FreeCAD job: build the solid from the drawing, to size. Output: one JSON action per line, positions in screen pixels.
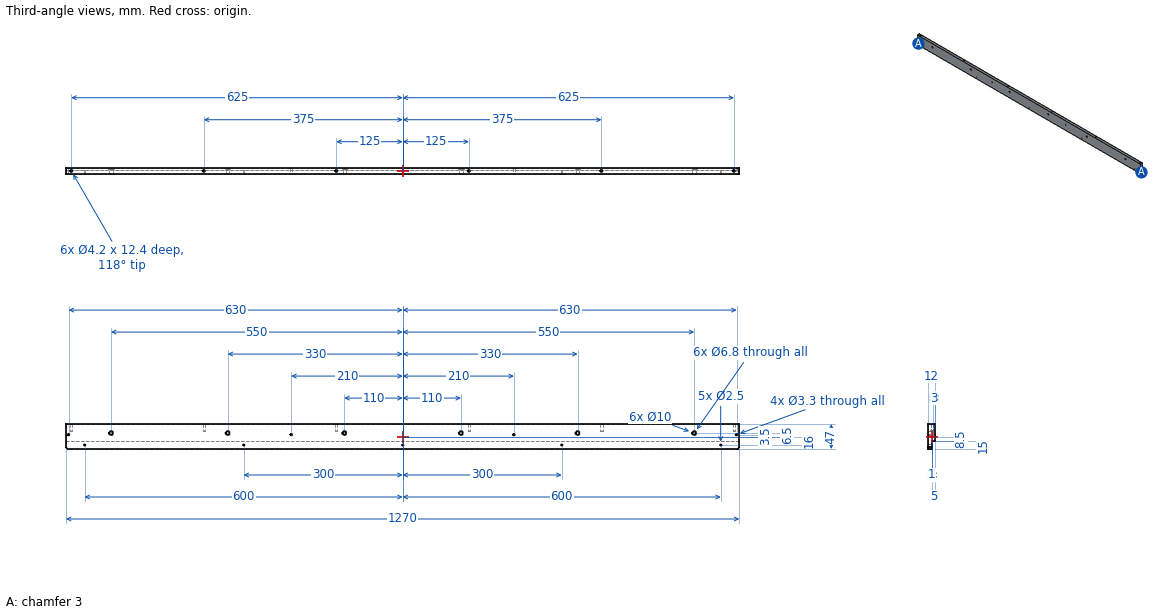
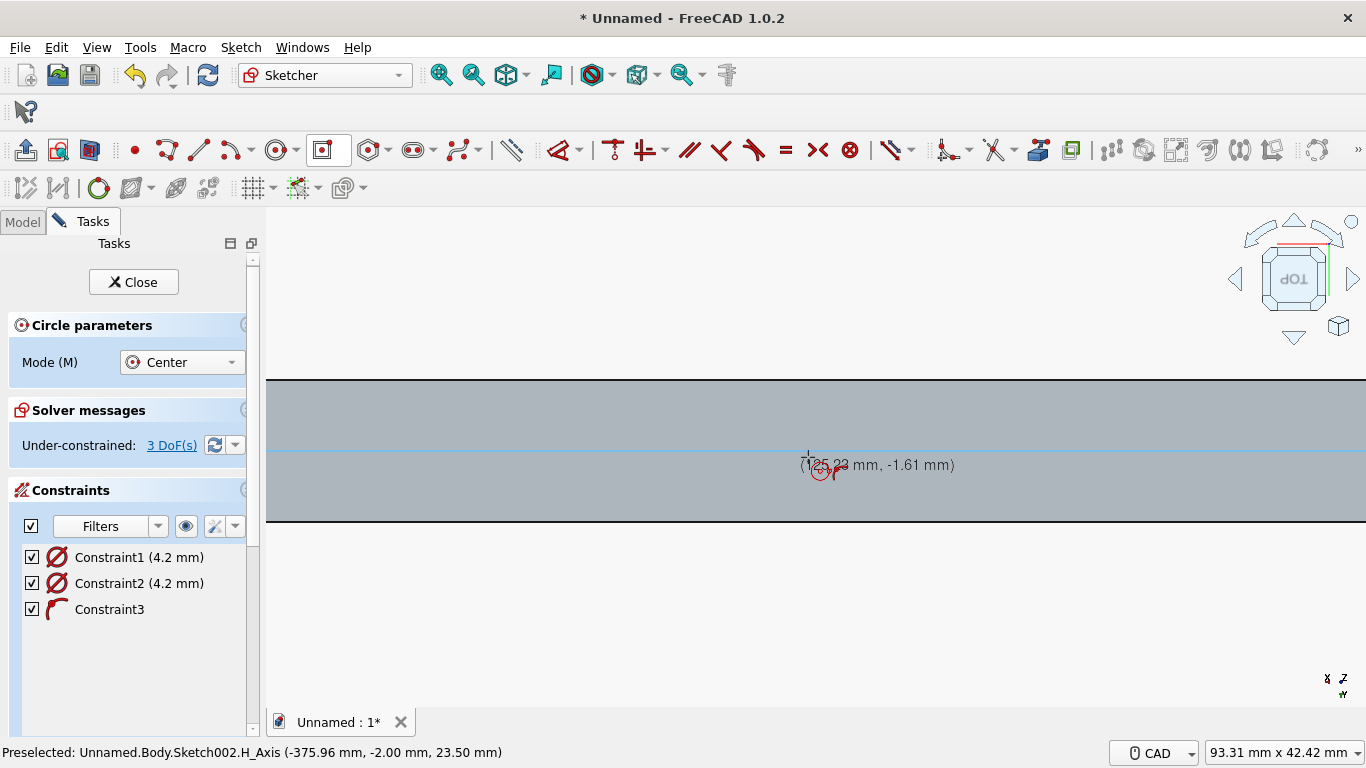
{"action": "scroll", "coordinate": [822, 457], "scroll_direction": "down", "scroll_amount": 15}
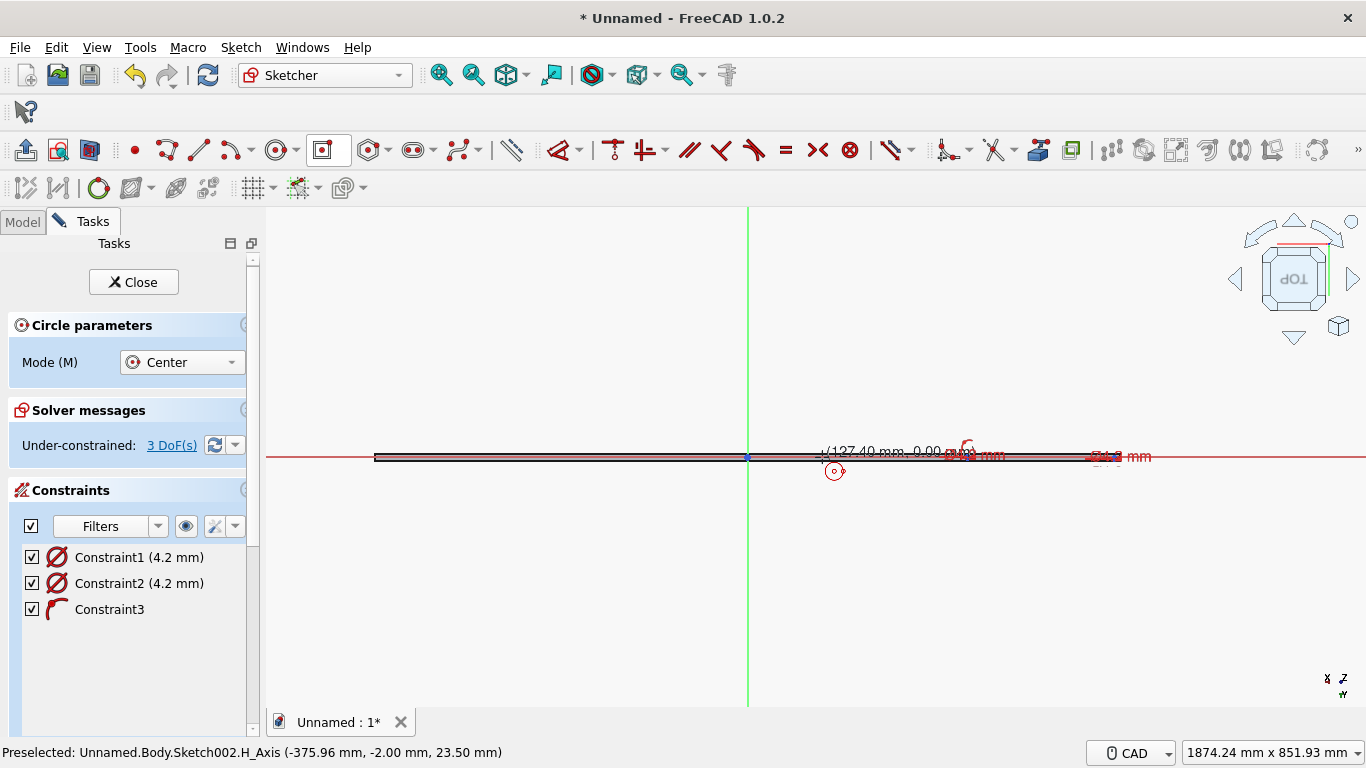
{"action": "left_click", "coordinate": [821, 457]}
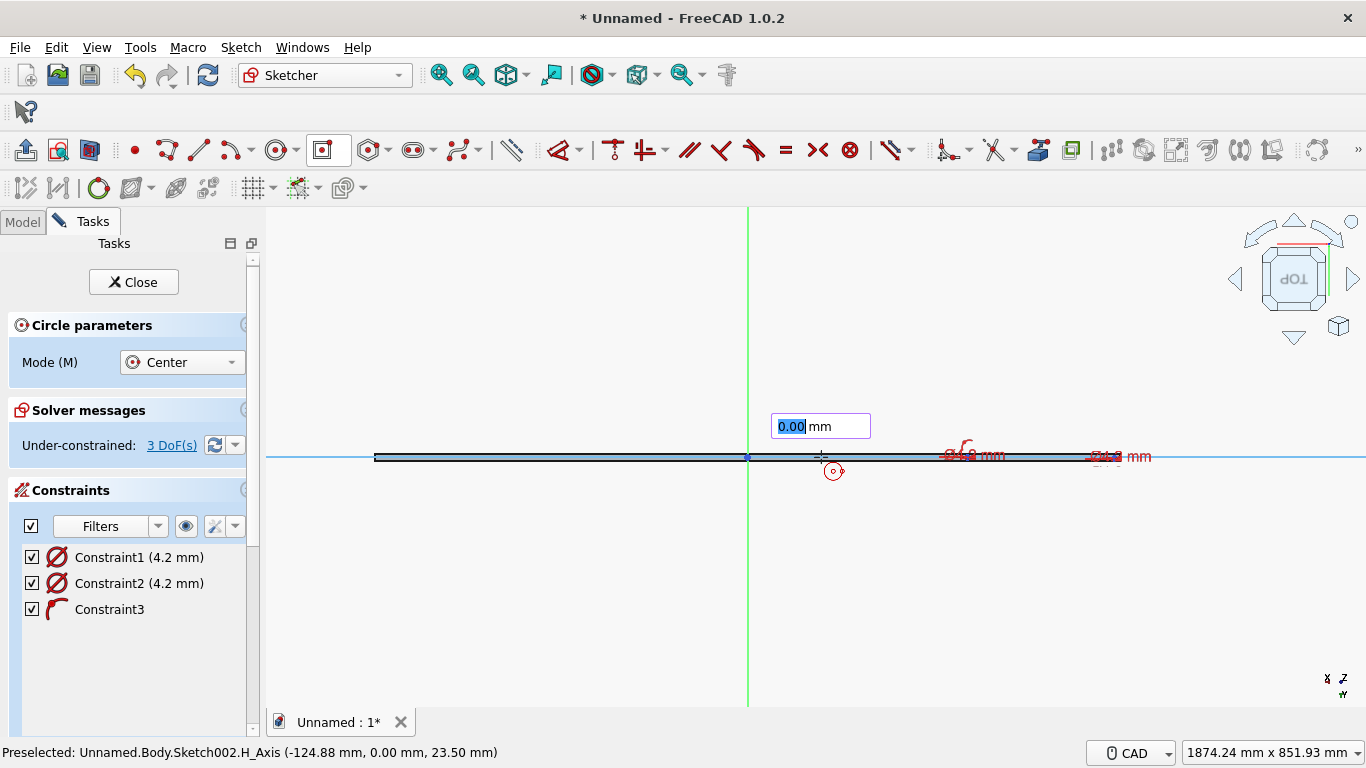
{"action": "scroll", "coordinate": [821, 458], "scroll_direction": "up", "scroll_amount": 14}
{"action": "mouse_move", "coordinate": [807, 456]}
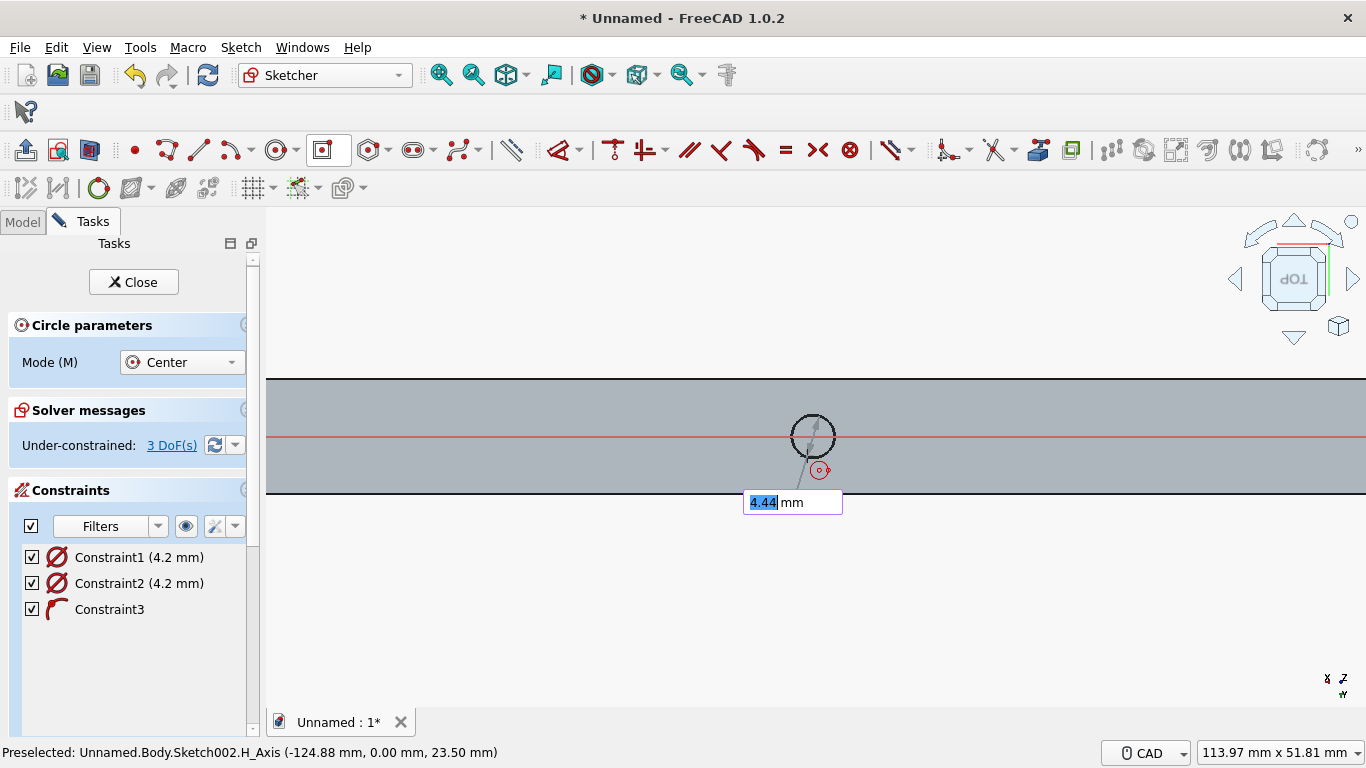
{"action": "type", "text": "4.2"}
{"action": "key", "text": "Return"}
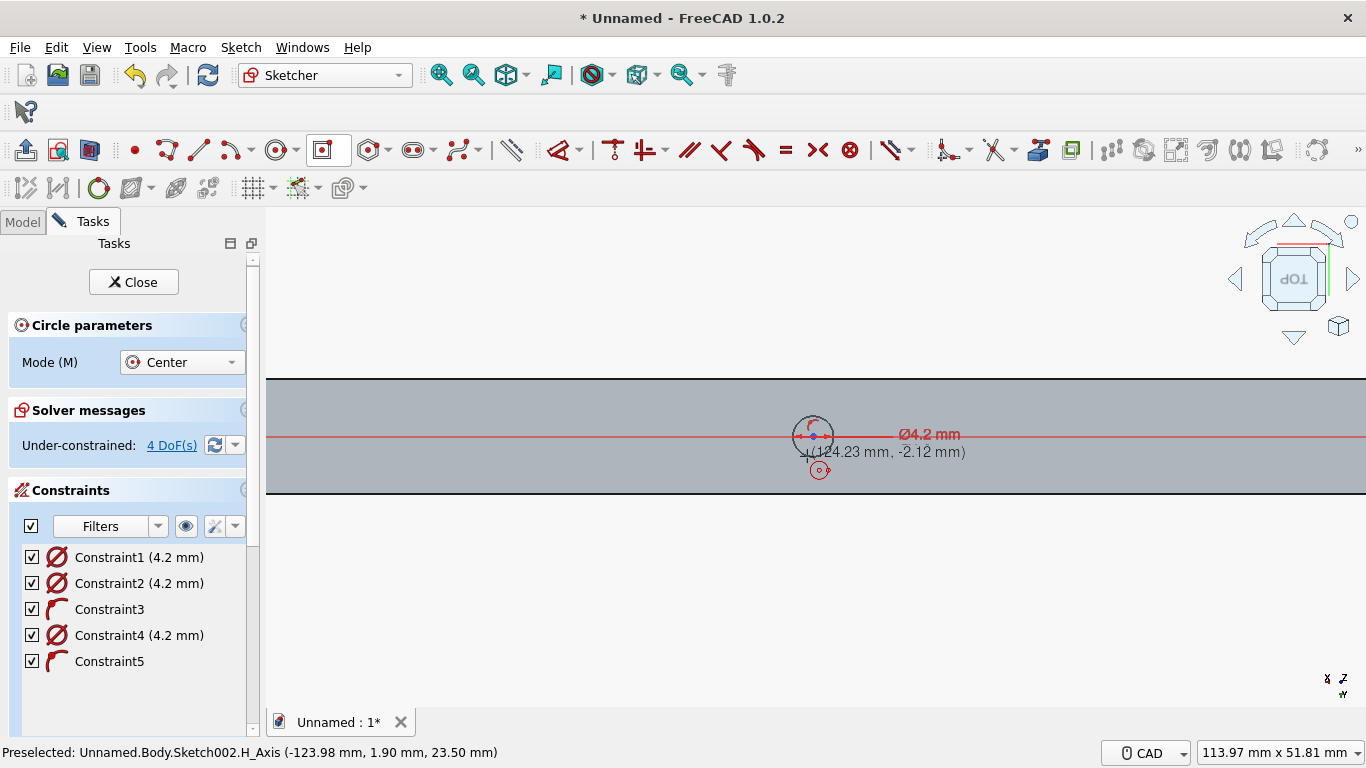
{"action": "scroll", "coordinate": [807, 458], "scroll_direction": "down", "scroll_amount": 15}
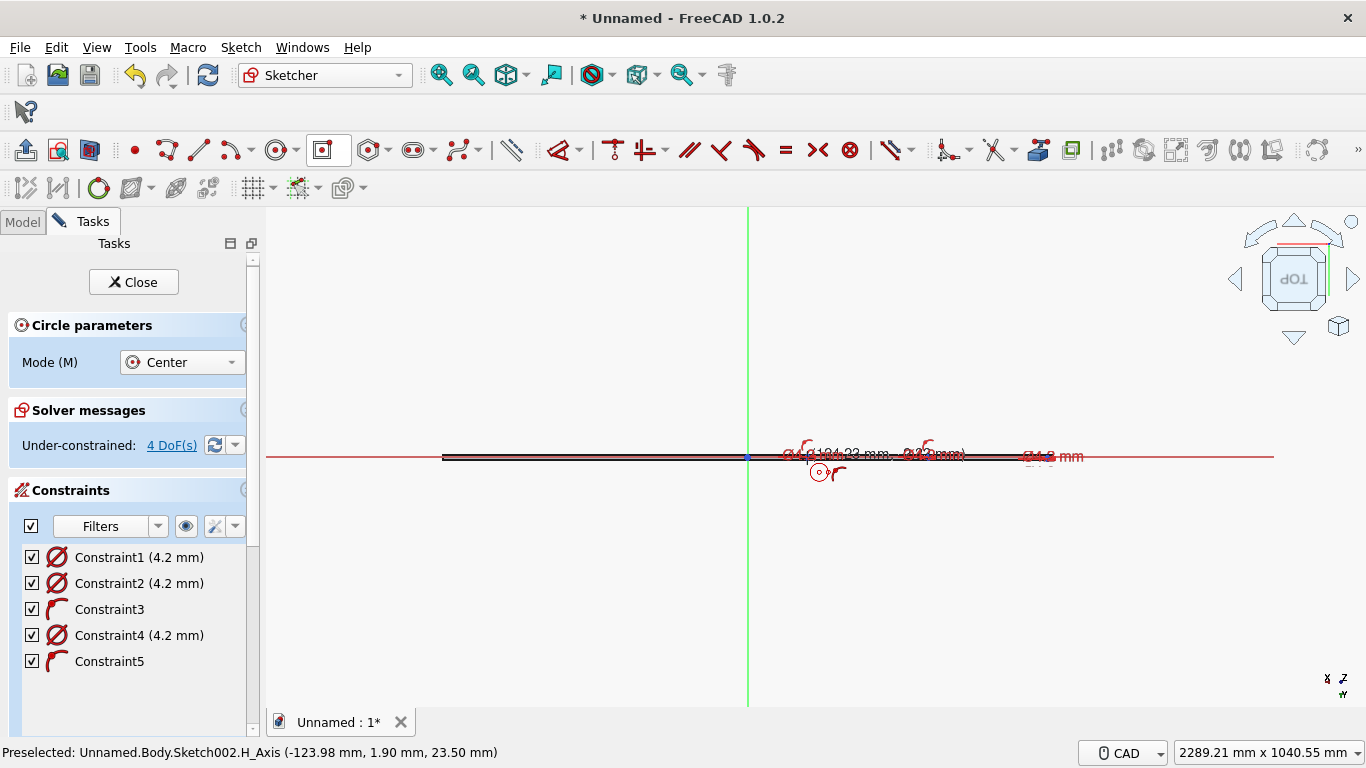
{"action": "scroll", "coordinate": [688, 457], "scroll_direction": "up", "scroll_amount": 16}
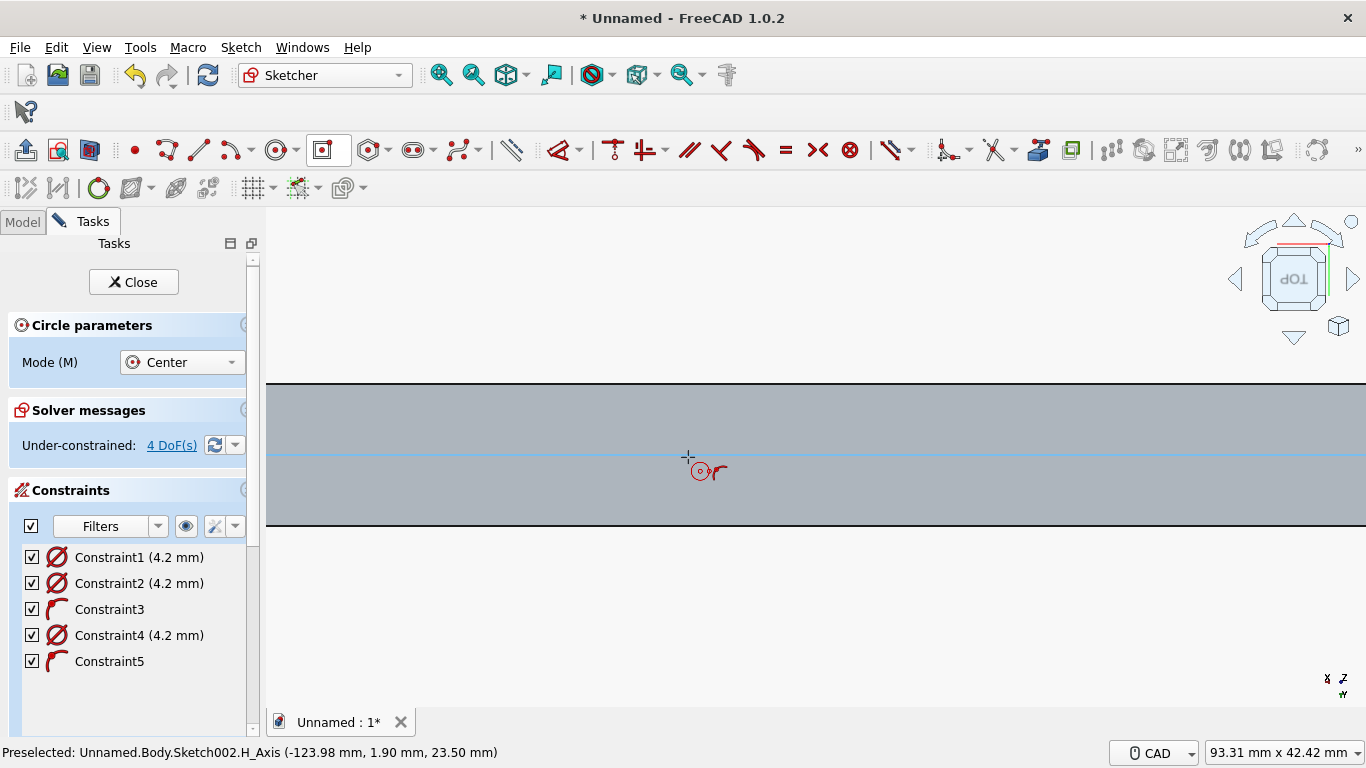
{"action": "scroll", "coordinate": [674, 457], "scroll_direction": "down", "scroll_amount": 15}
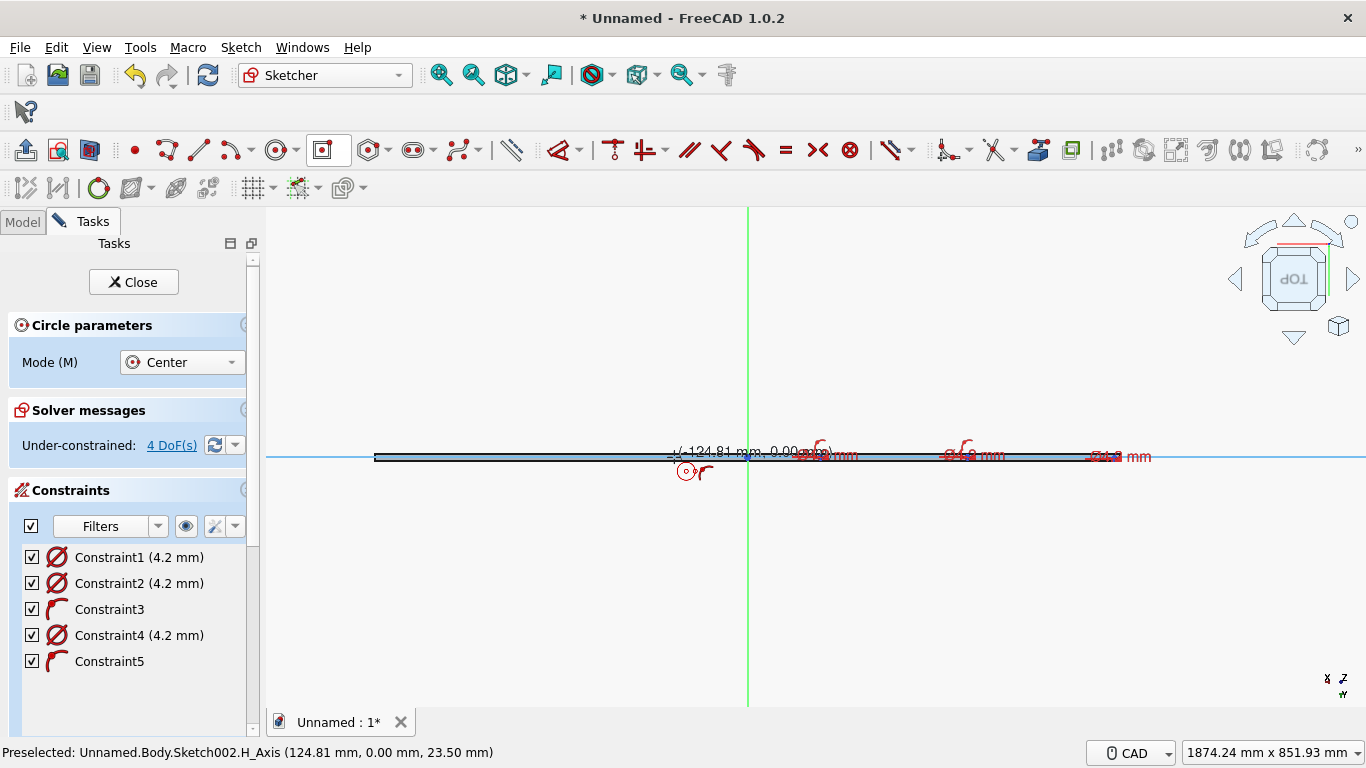
{"action": "left_click", "coordinate": [674, 457]}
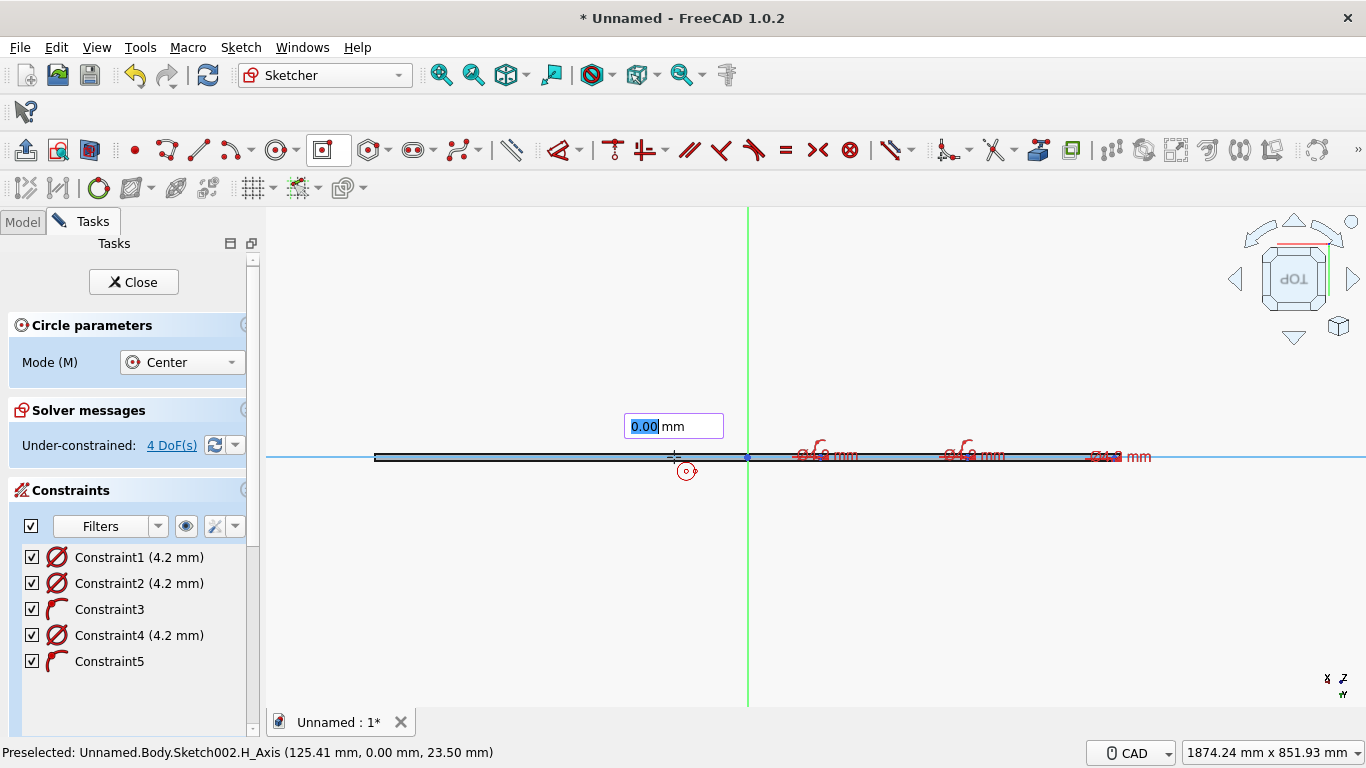
{"action": "scroll", "coordinate": [674, 459], "scroll_direction": "up", "scroll_amount": 14}
{"action": "mouse_move", "coordinate": [665, 444]}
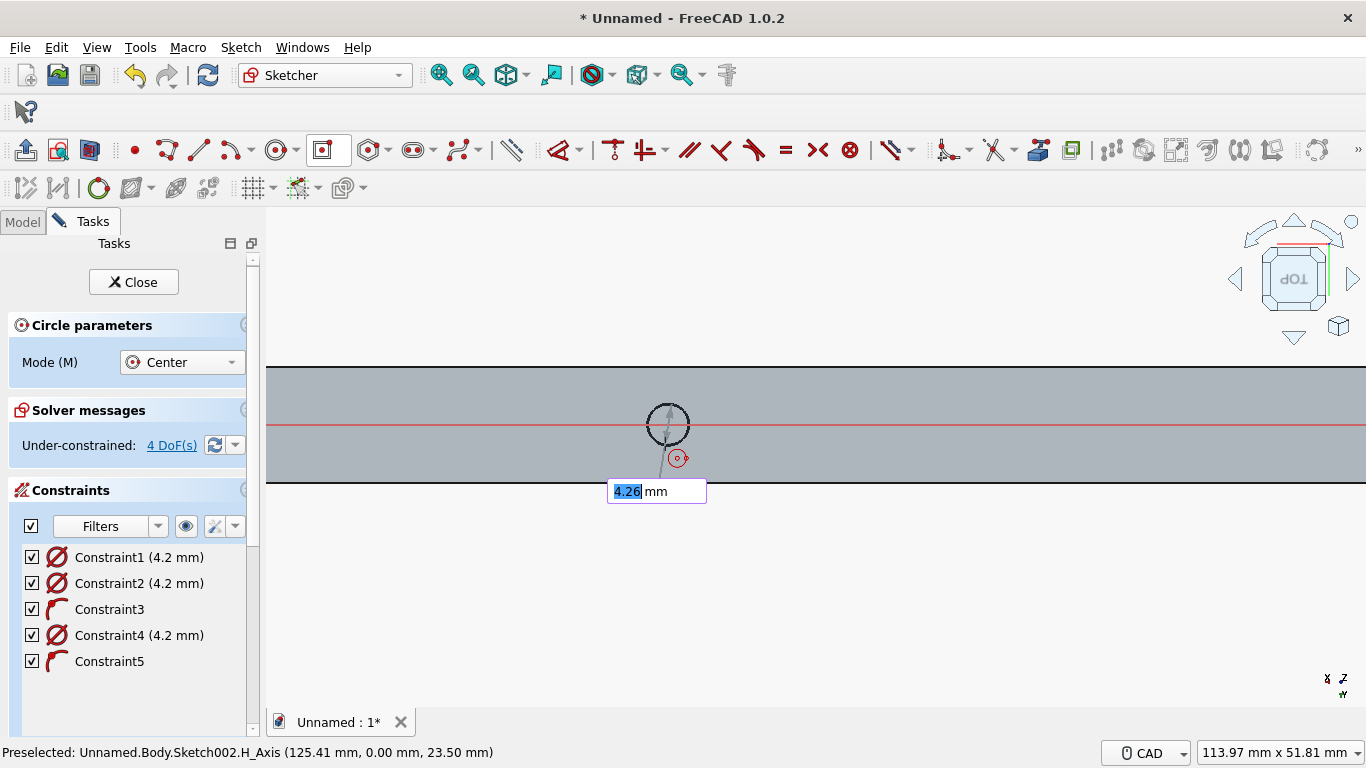
{"action": "type", "text": "4.2"}
{"action": "key", "text": "Return"}